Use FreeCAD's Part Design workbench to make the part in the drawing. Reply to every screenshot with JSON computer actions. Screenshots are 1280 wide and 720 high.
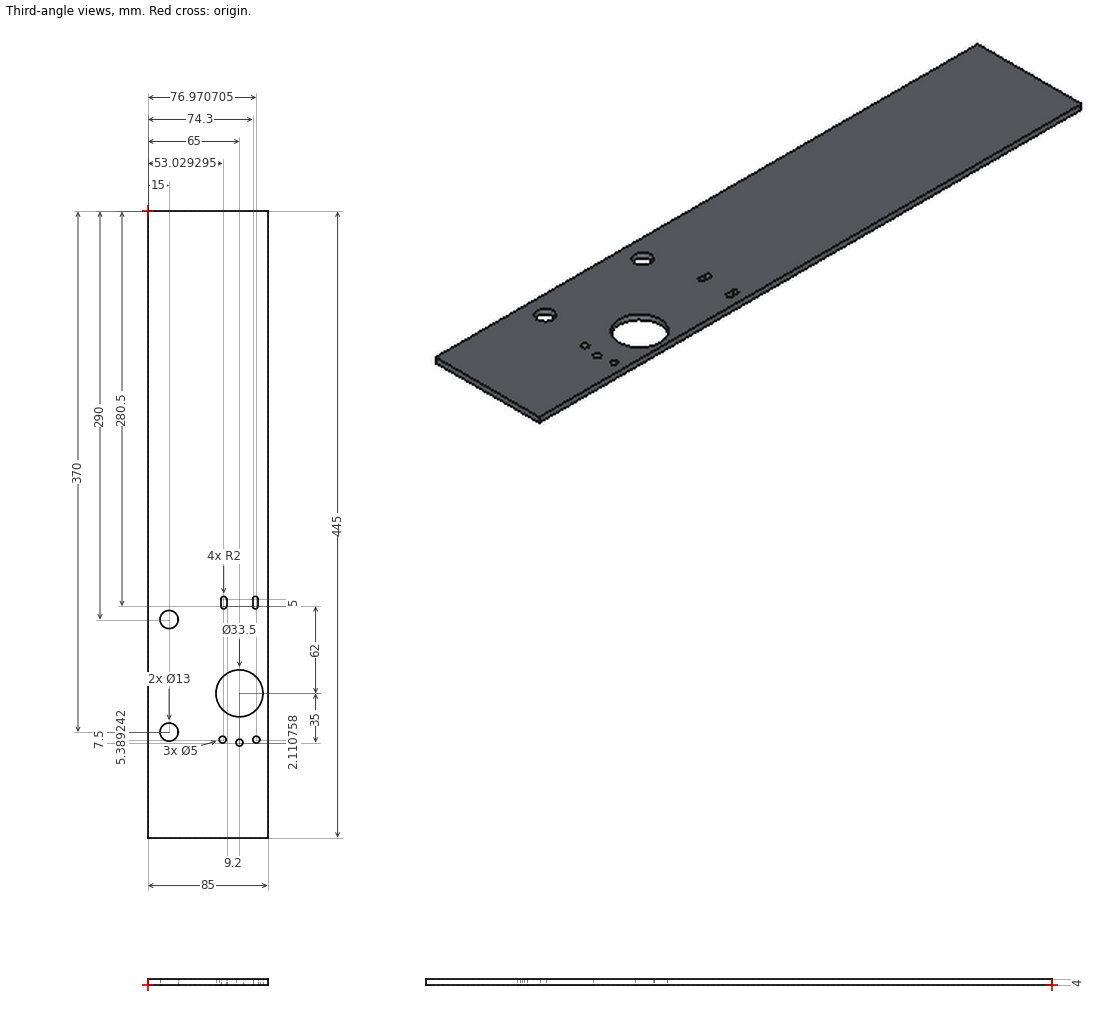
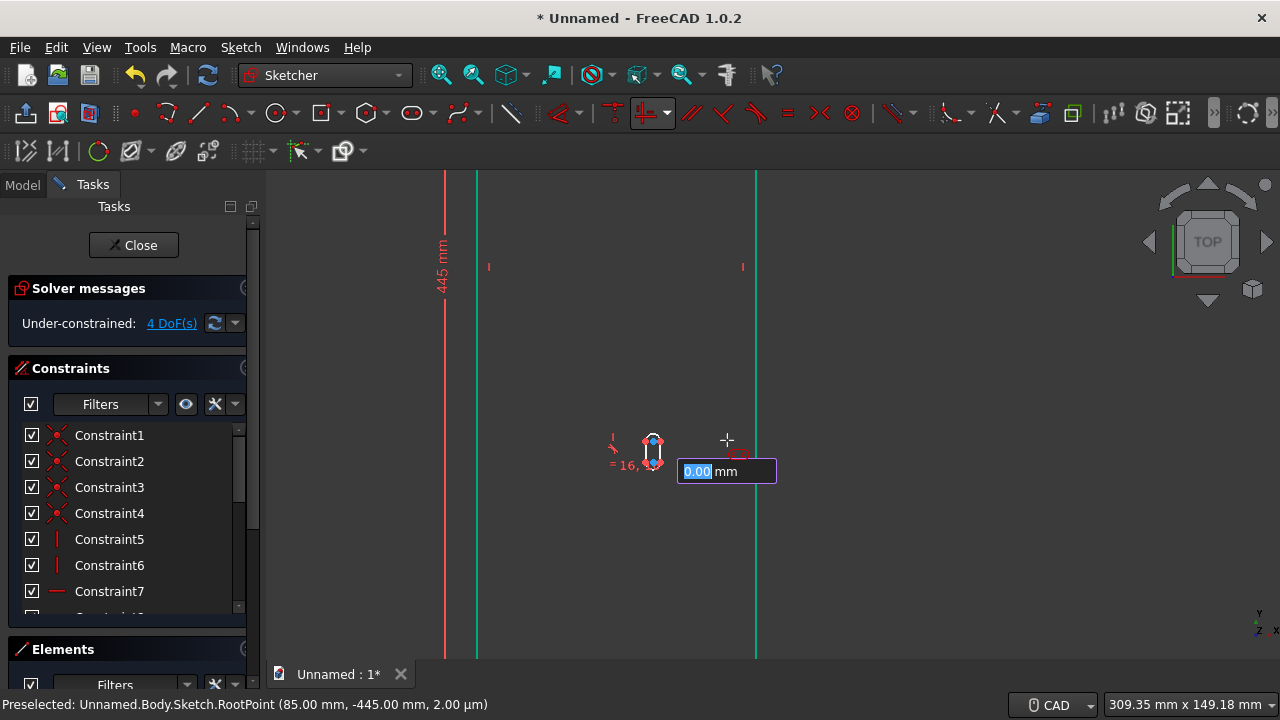
{"action": "scroll", "coordinate": [734, 448], "scroll_direction": "up", "scroll_amount": 5}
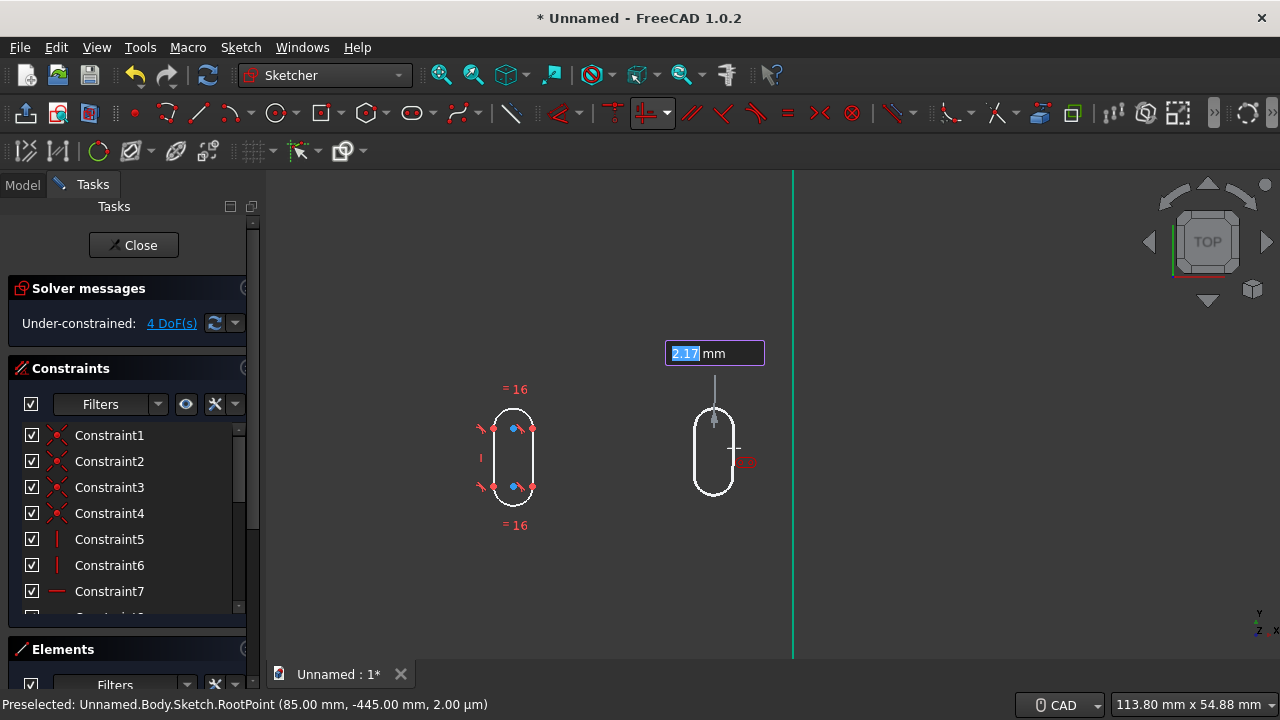
{"action": "left_click", "coordinate": [733, 448]}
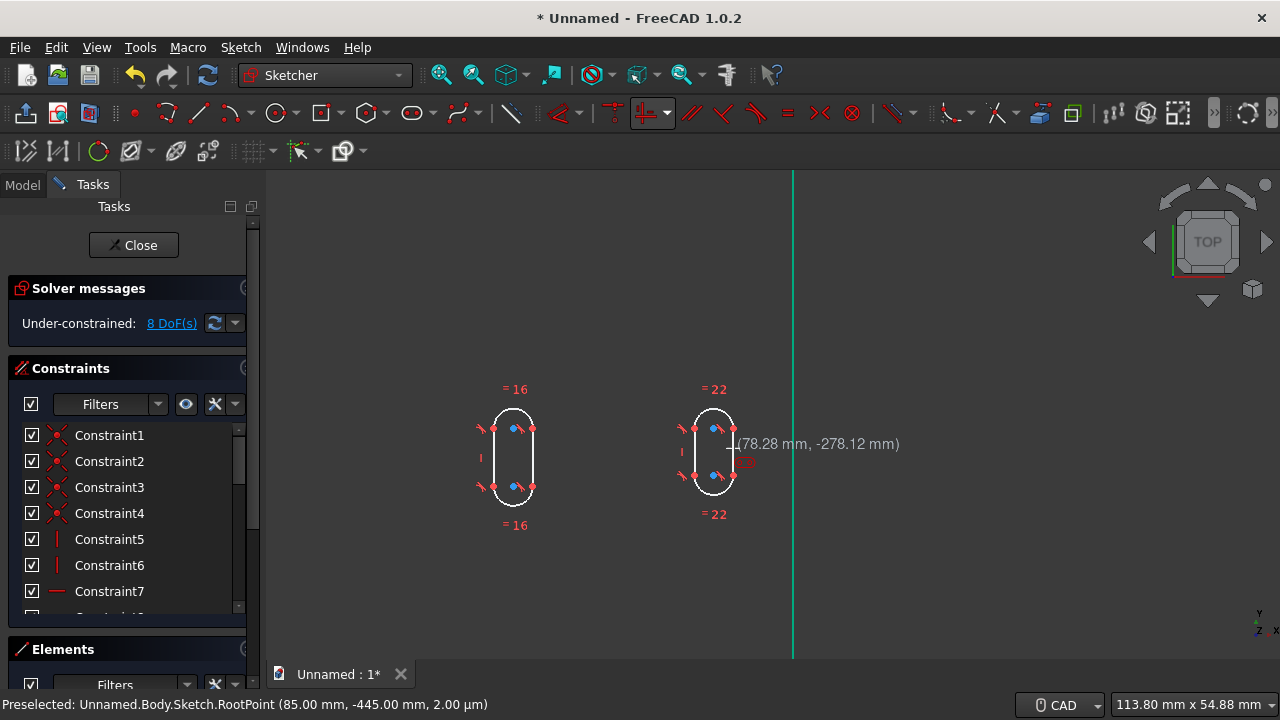
{"action": "key", "text": "g c"}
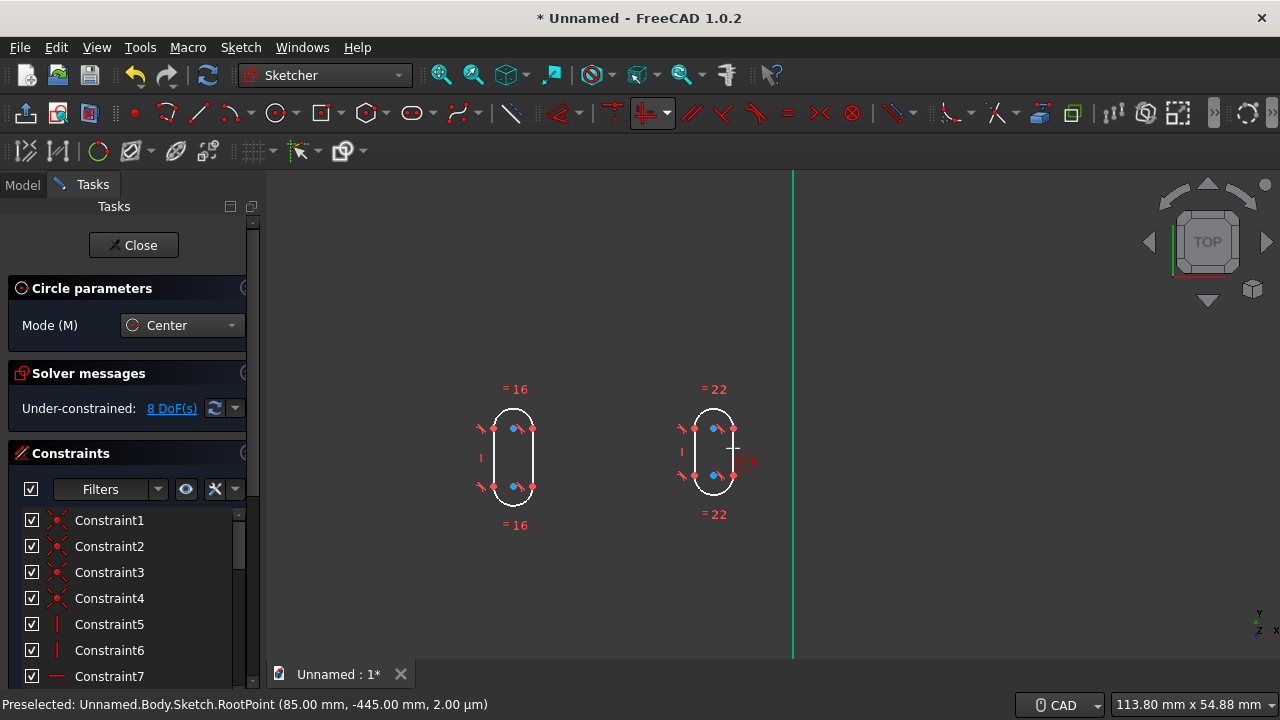
{"action": "scroll", "coordinate": [728, 451], "scroll_direction": "down", "scroll_amount": 13}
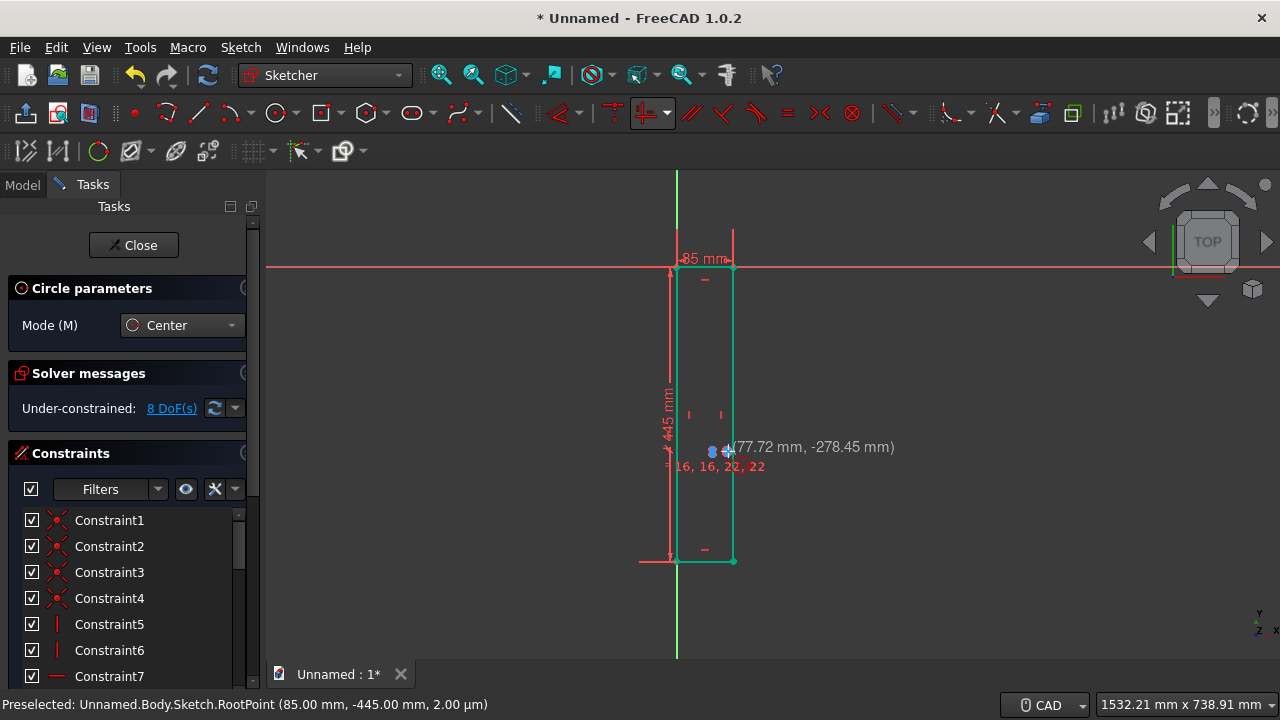
{"action": "scroll", "coordinate": [687, 512], "scroll_direction": "up", "scroll_amount": 9}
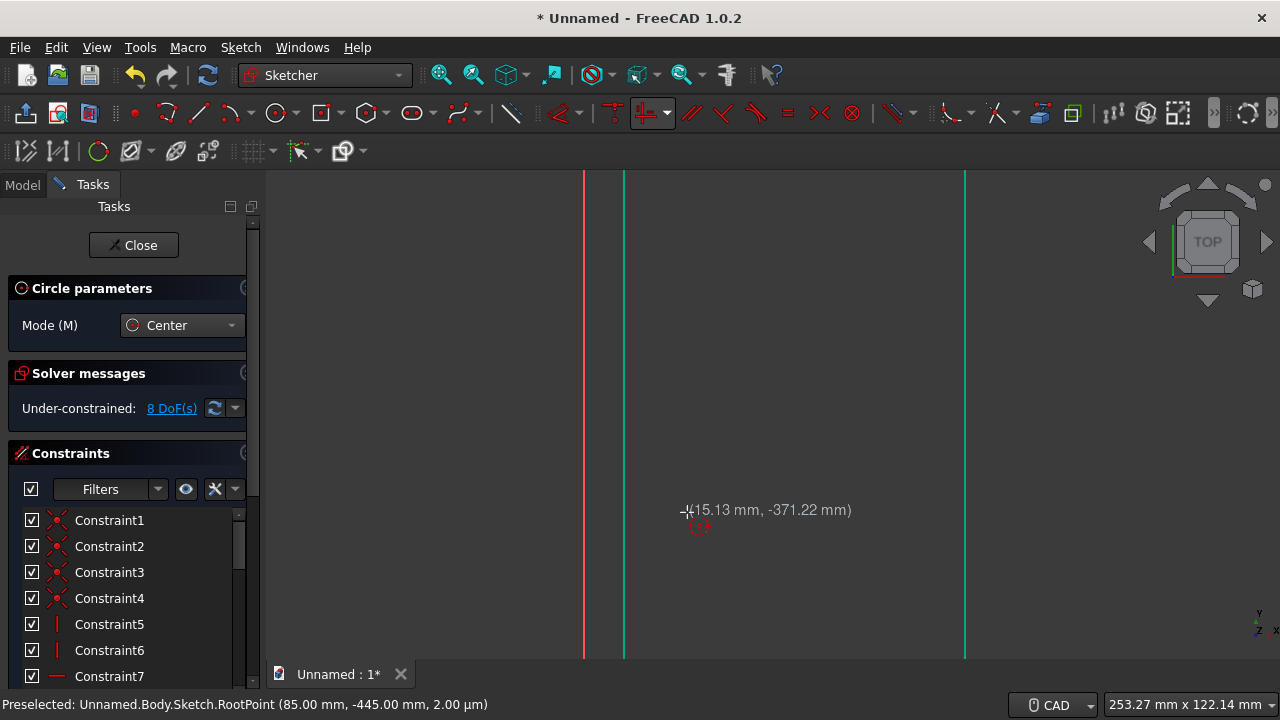
{"action": "scroll", "coordinate": [687, 513], "scroll_direction": "down", "scroll_amount": 9}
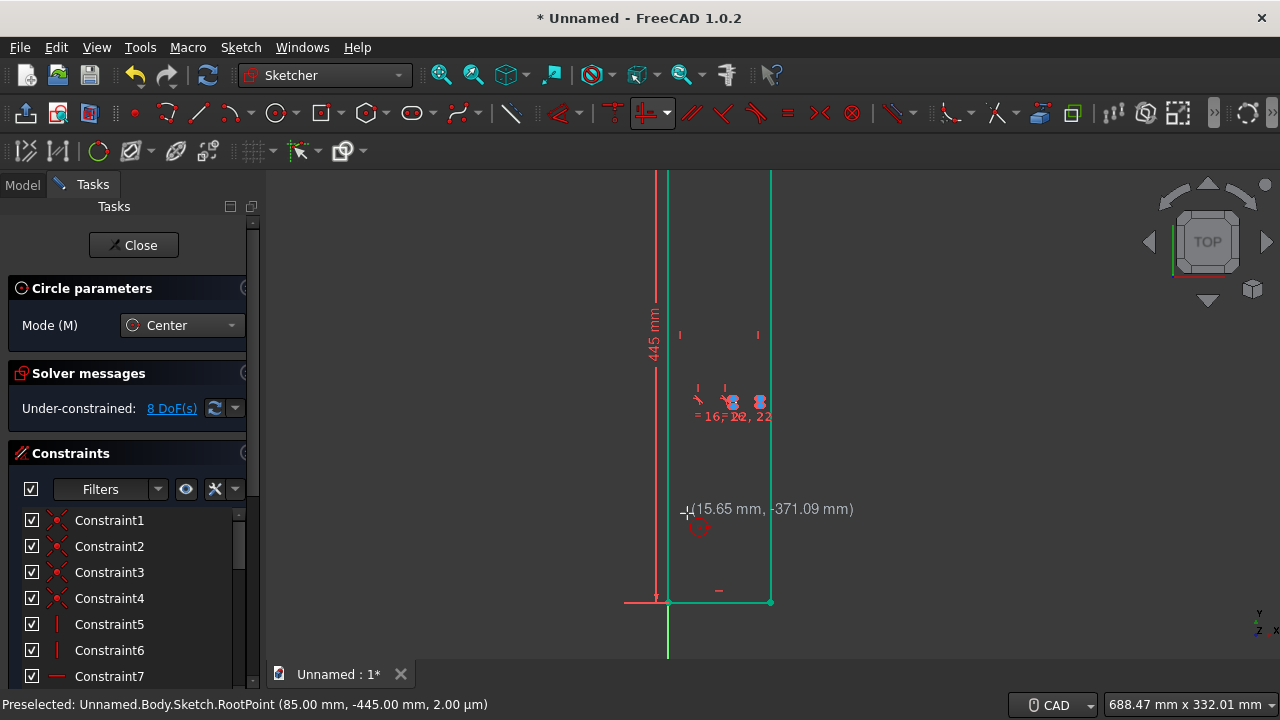
{"action": "scroll", "coordinate": [687, 513], "scroll_direction": "up", "scroll_amount": 3}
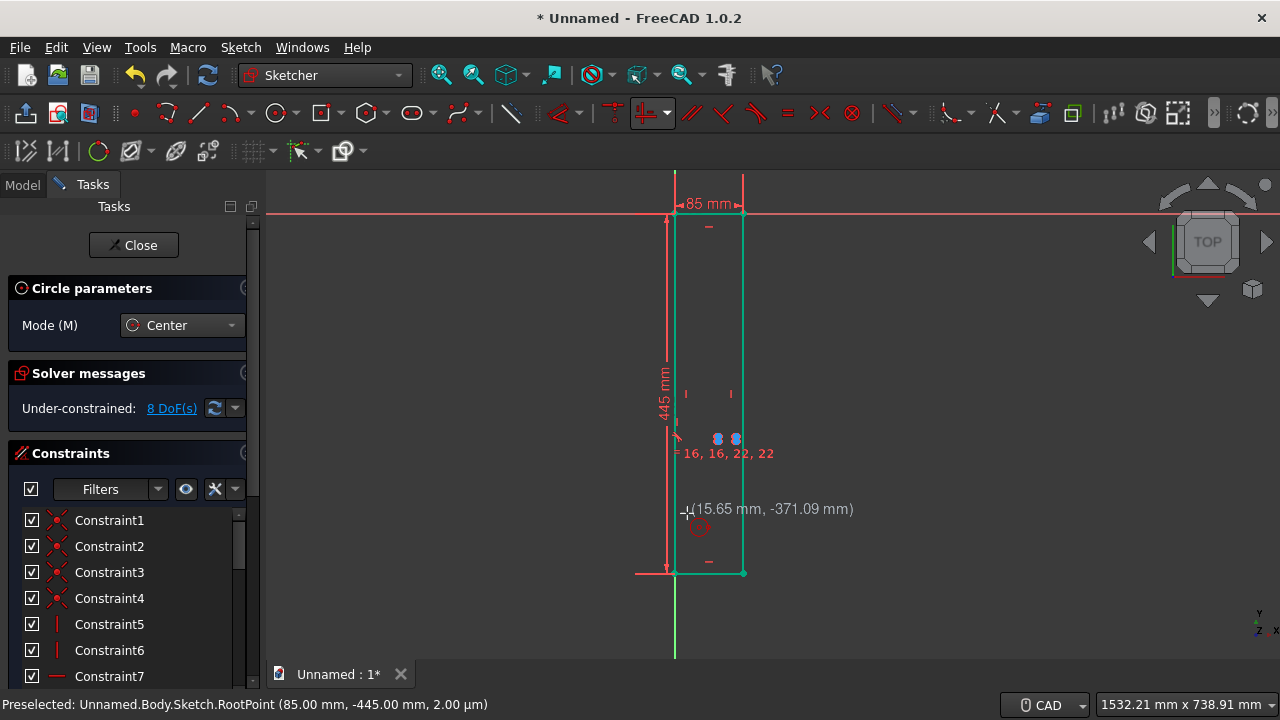
{"action": "left_click", "coordinate": [687, 512]}
{"action": "mouse_move", "coordinate": [692, 507]}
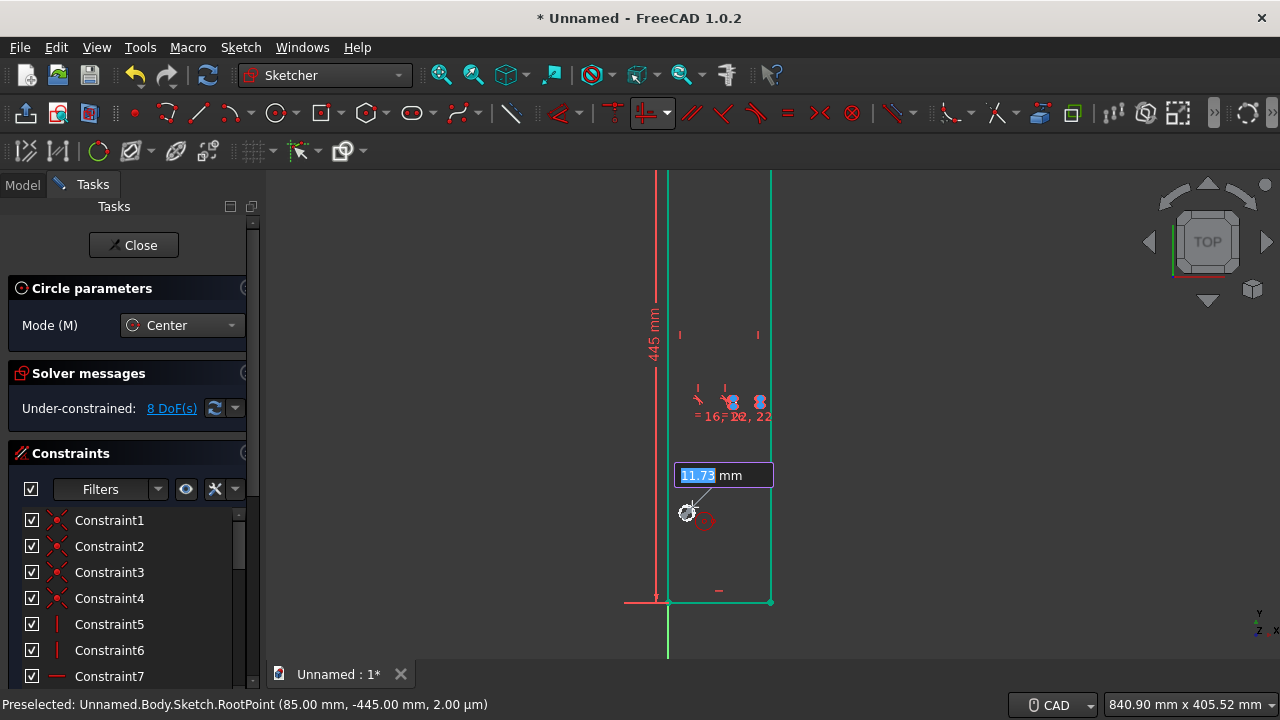
{"action": "type", "text": "13"}
{"action": "key", "text": "Return"}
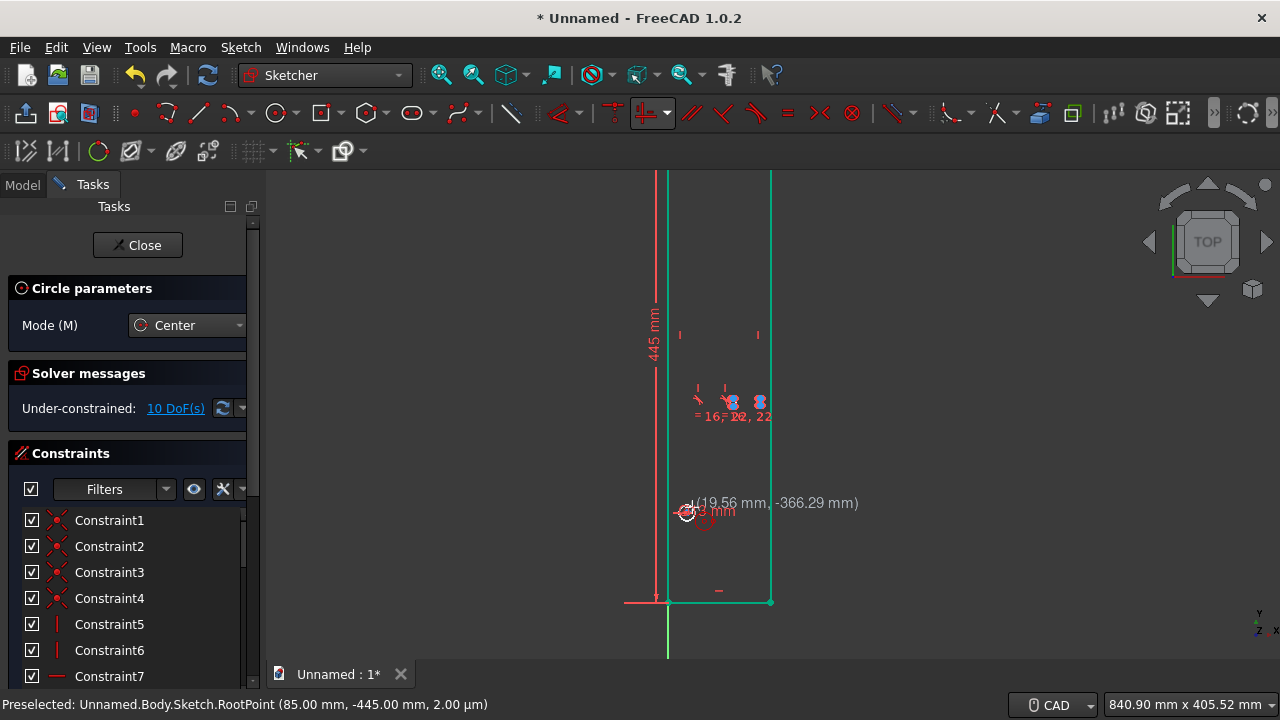
{"action": "scroll", "coordinate": [732, 519], "scroll_direction": "up", "scroll_amount": 11}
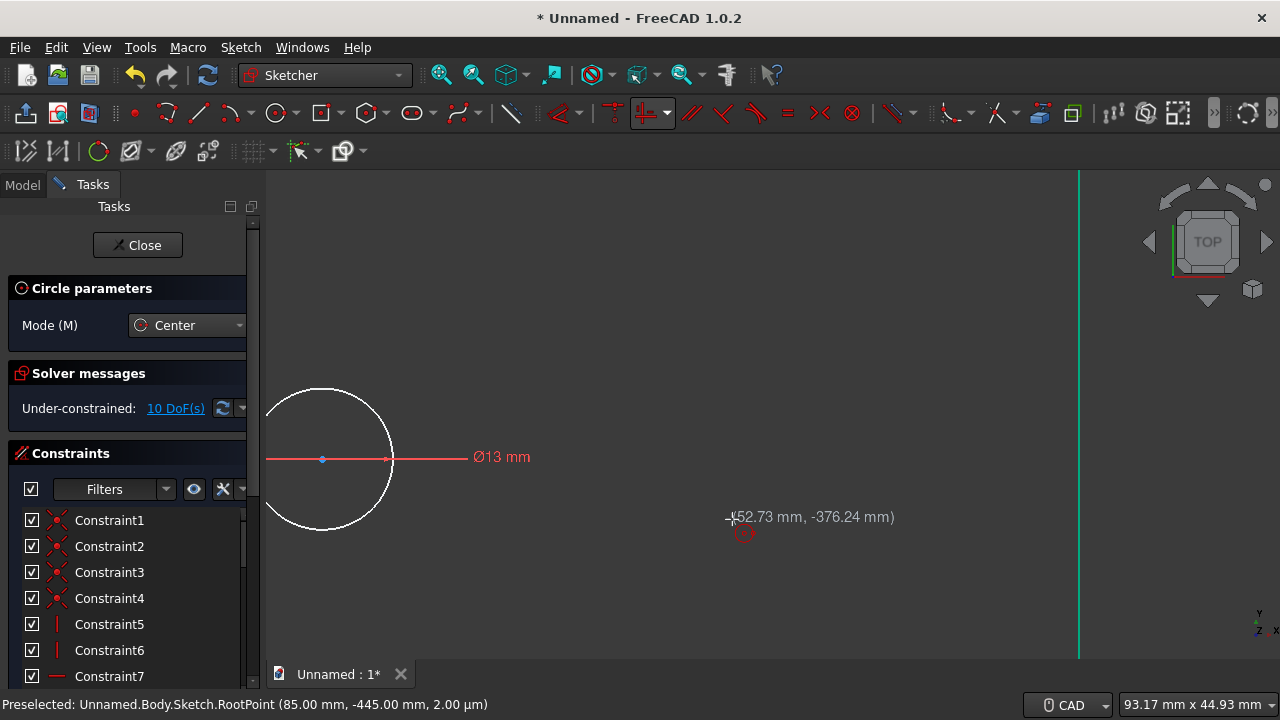
{"action": "scroll", "coordinate": [710, 516], "scroll_direction": "down", "scroll_amount": 14}